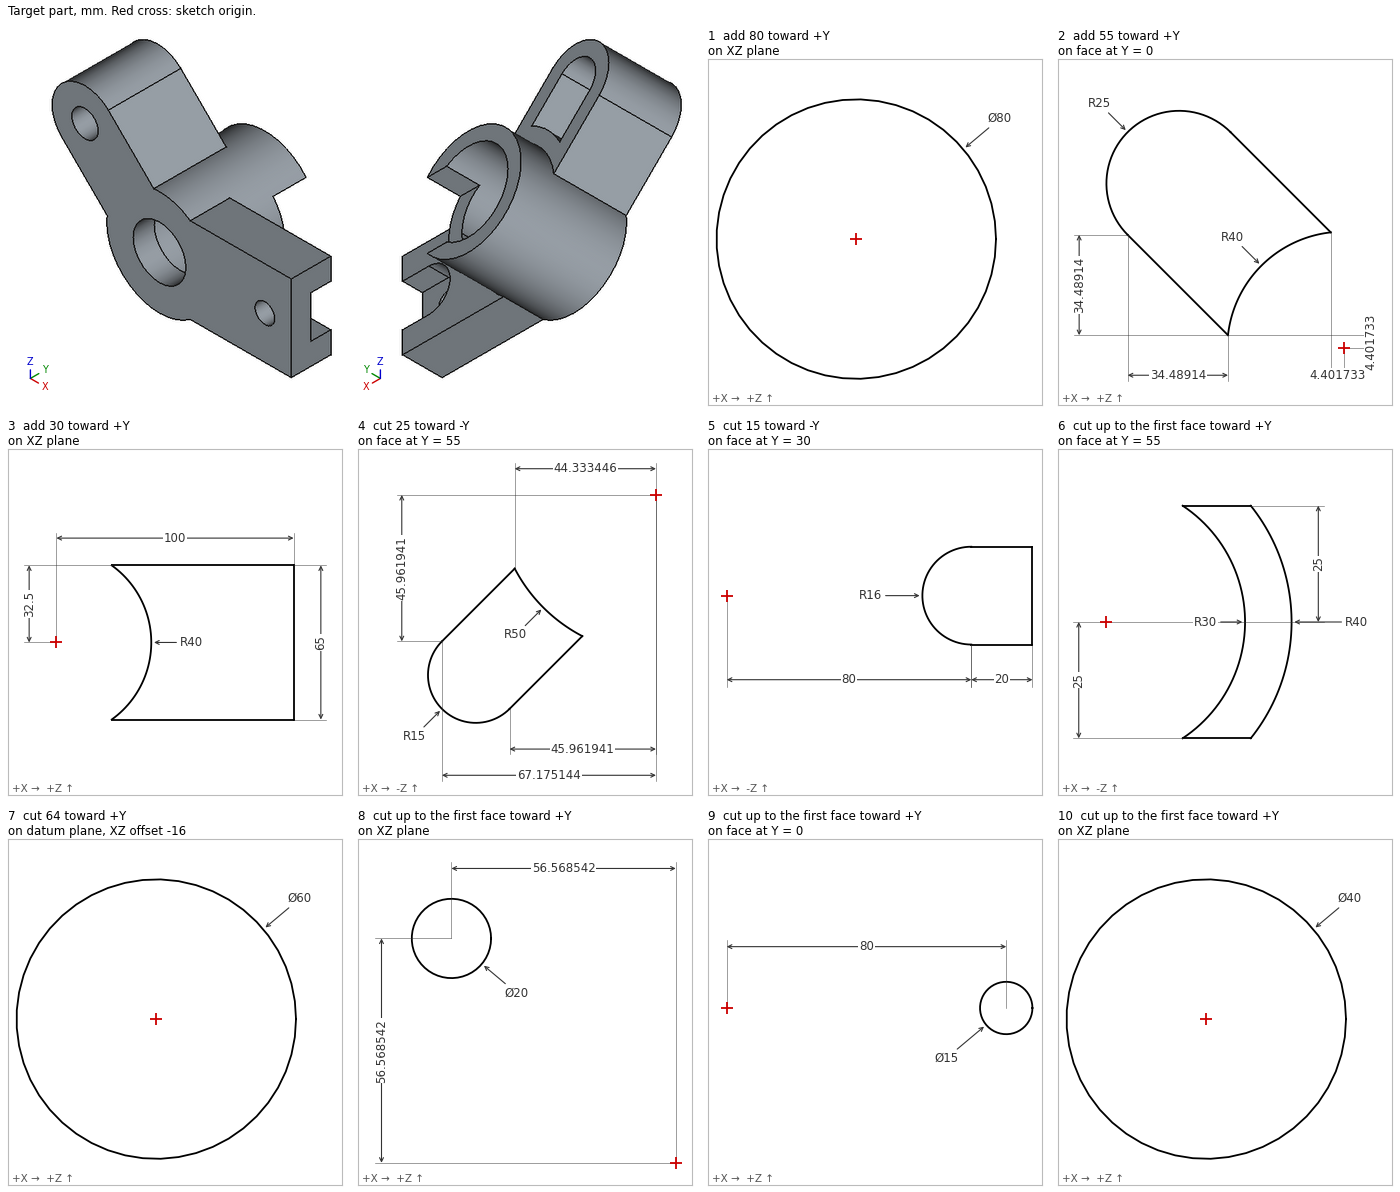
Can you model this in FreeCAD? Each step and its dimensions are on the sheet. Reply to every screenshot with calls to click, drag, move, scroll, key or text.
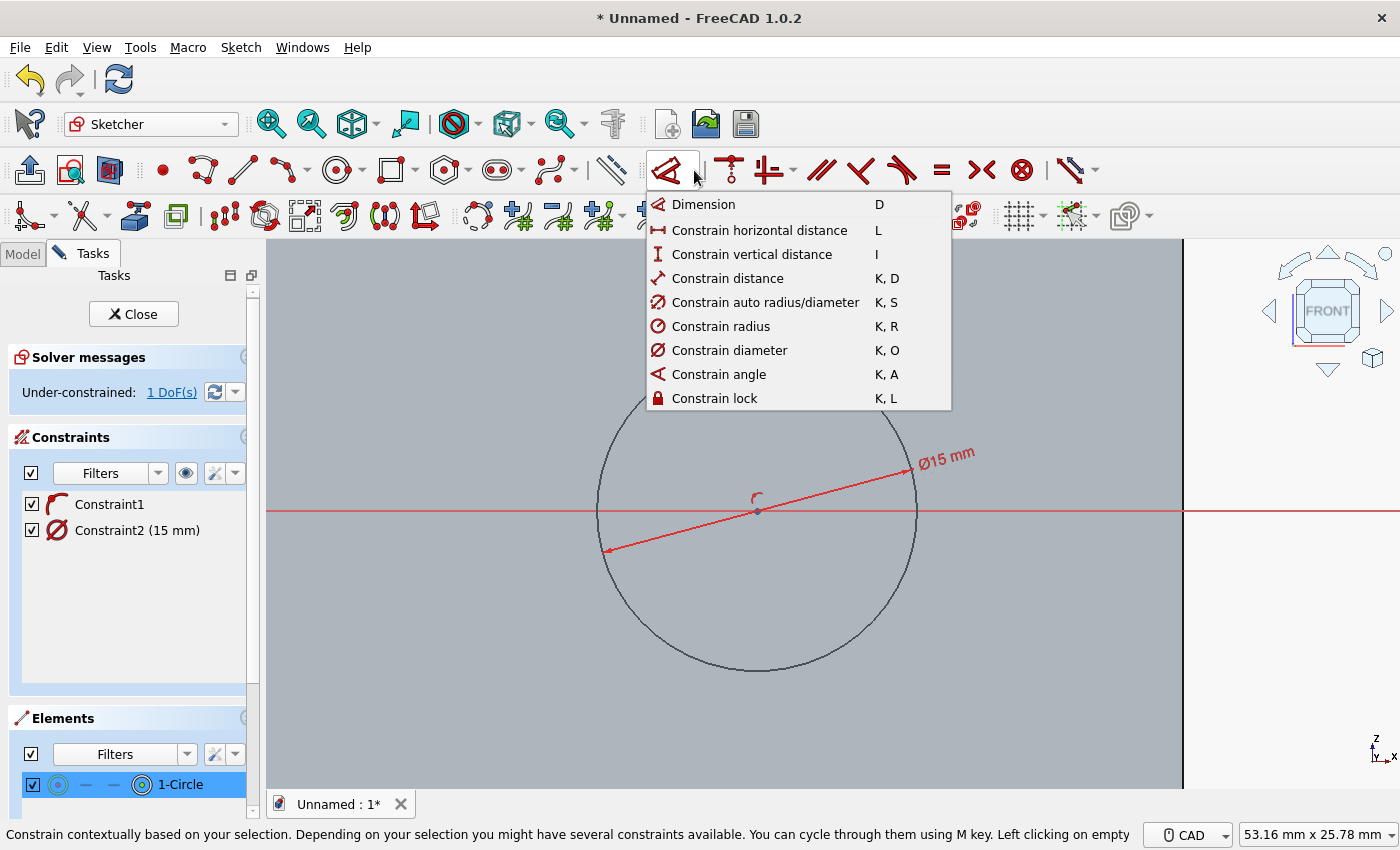
click(799, 230)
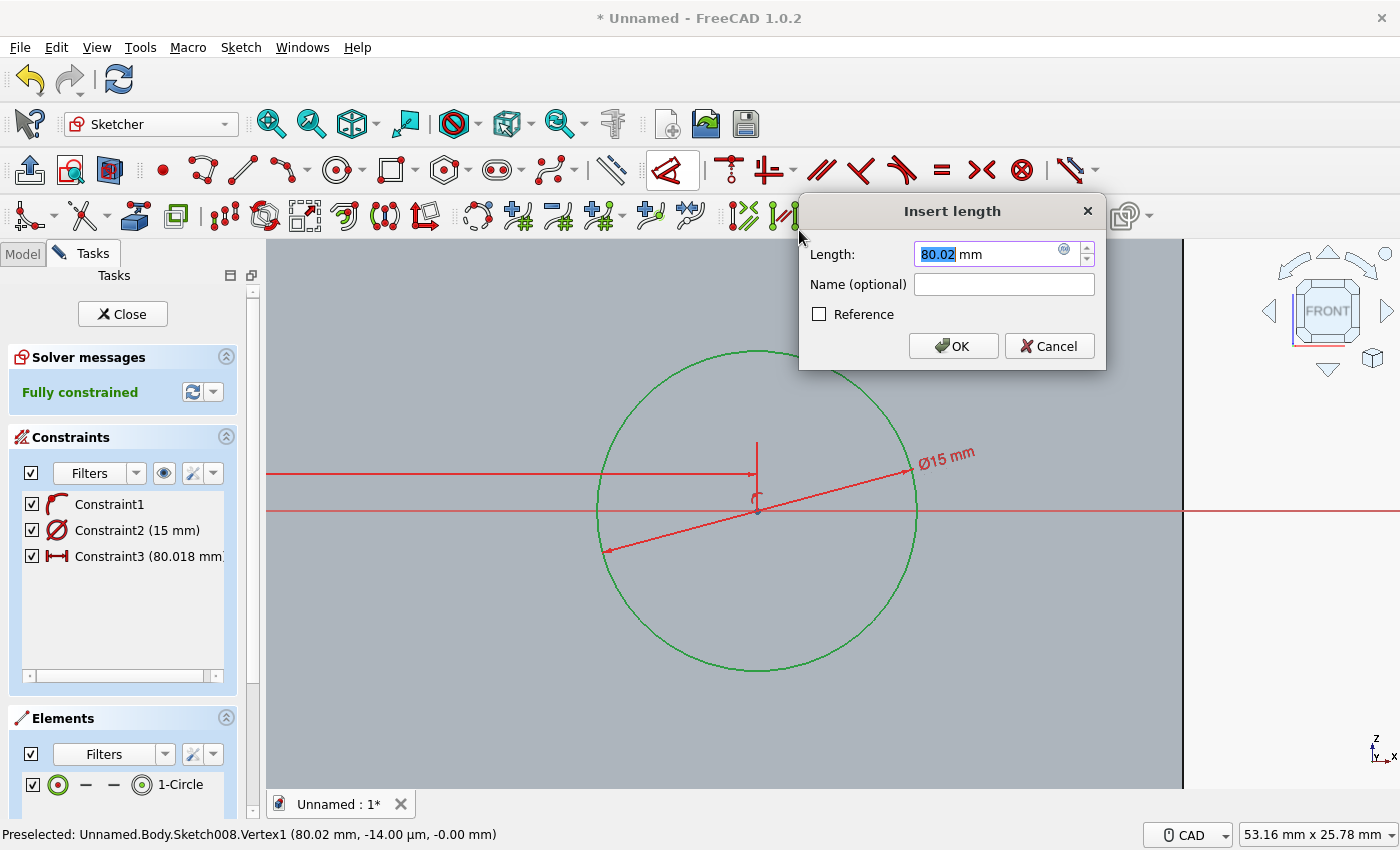
text(80)
key(Return)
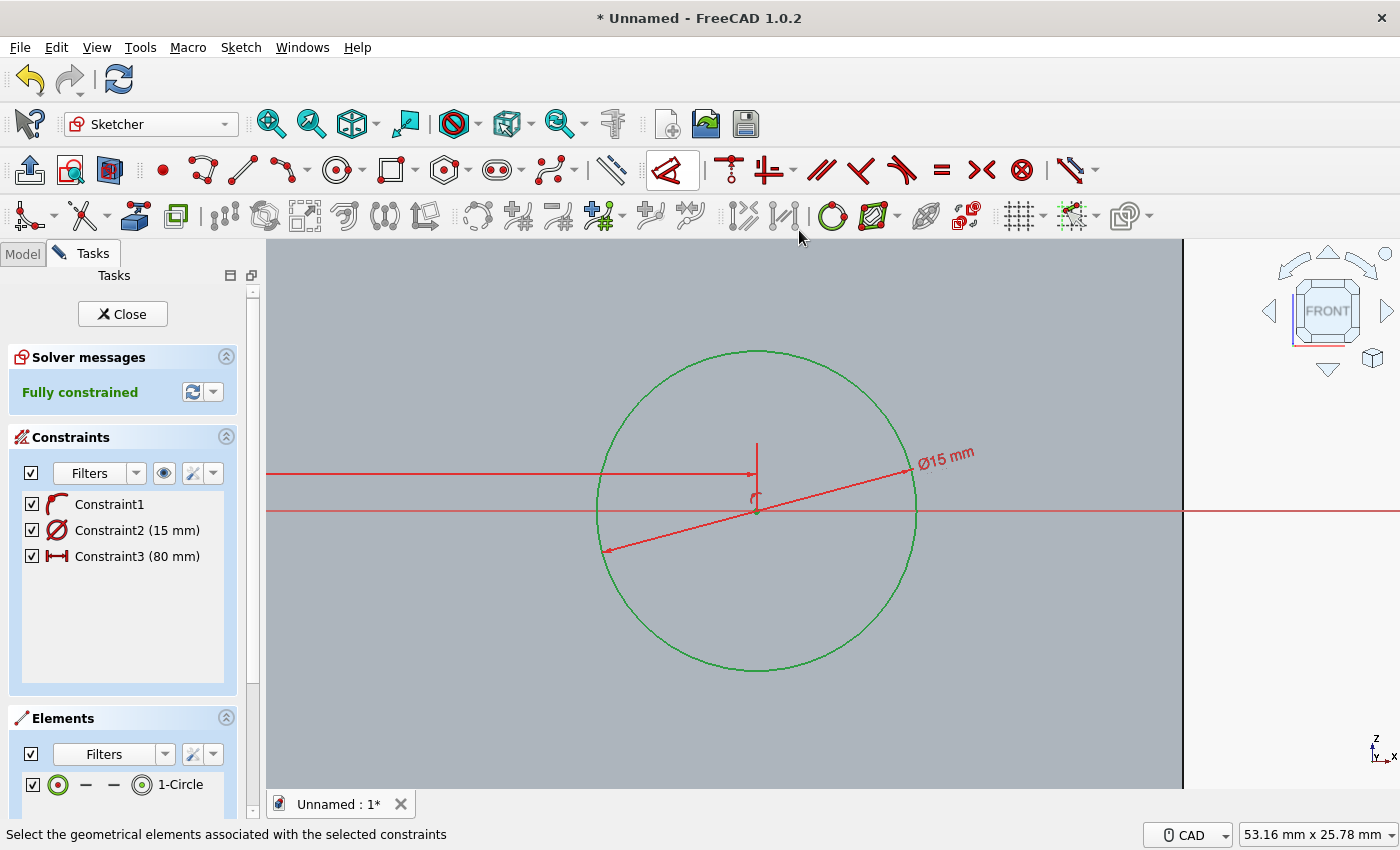
click(123, 314)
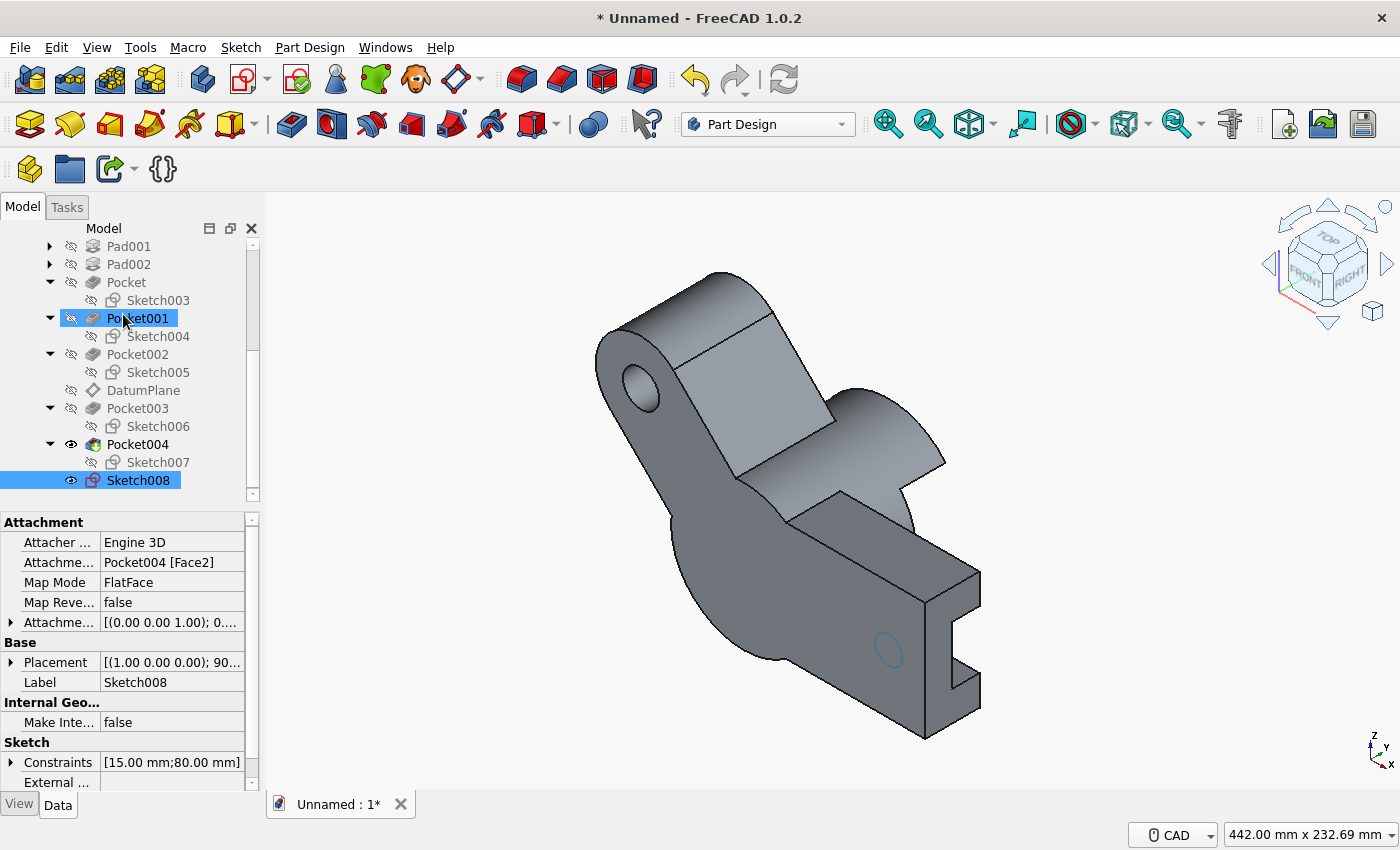
click(292, 124)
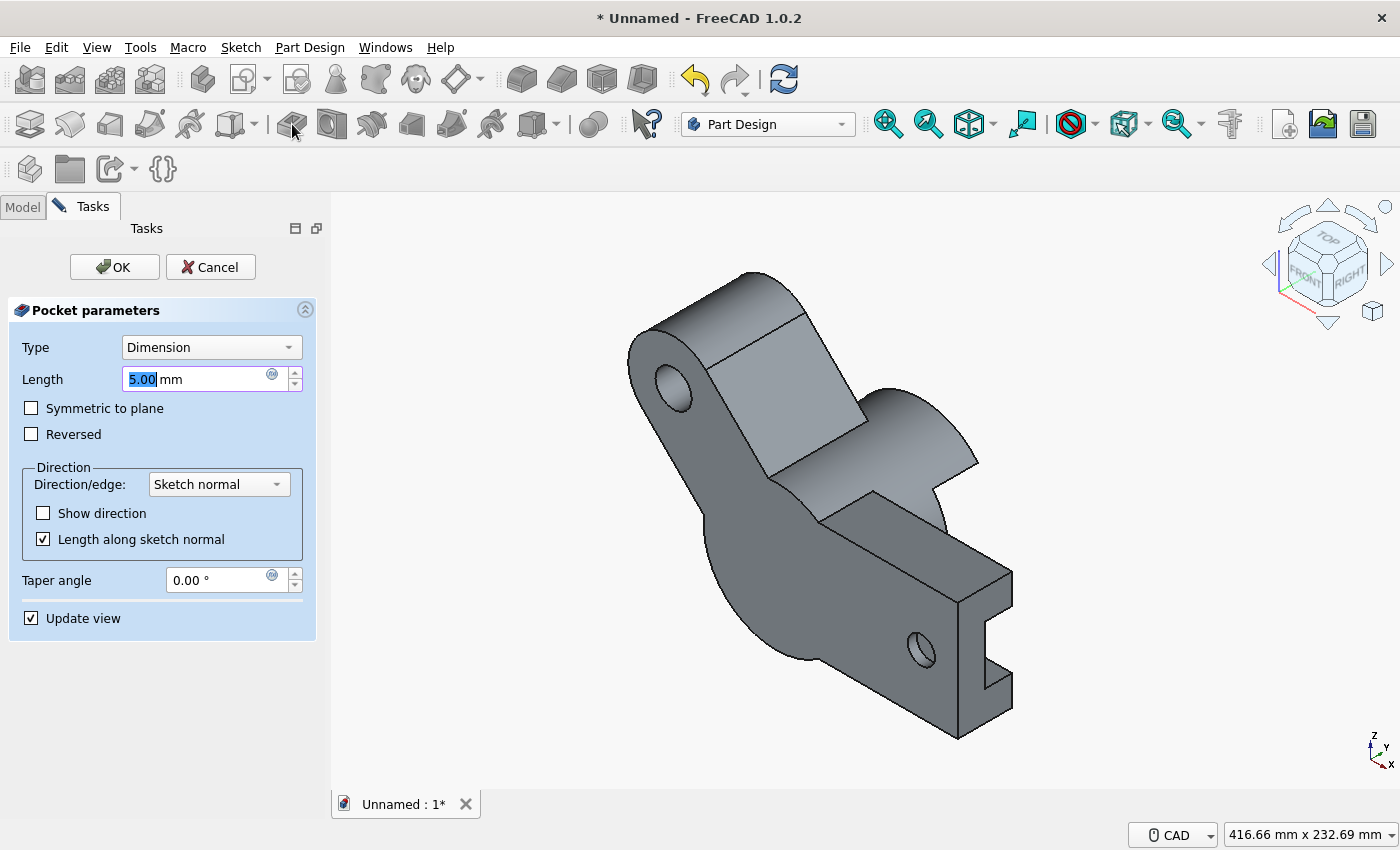
click(212, 348)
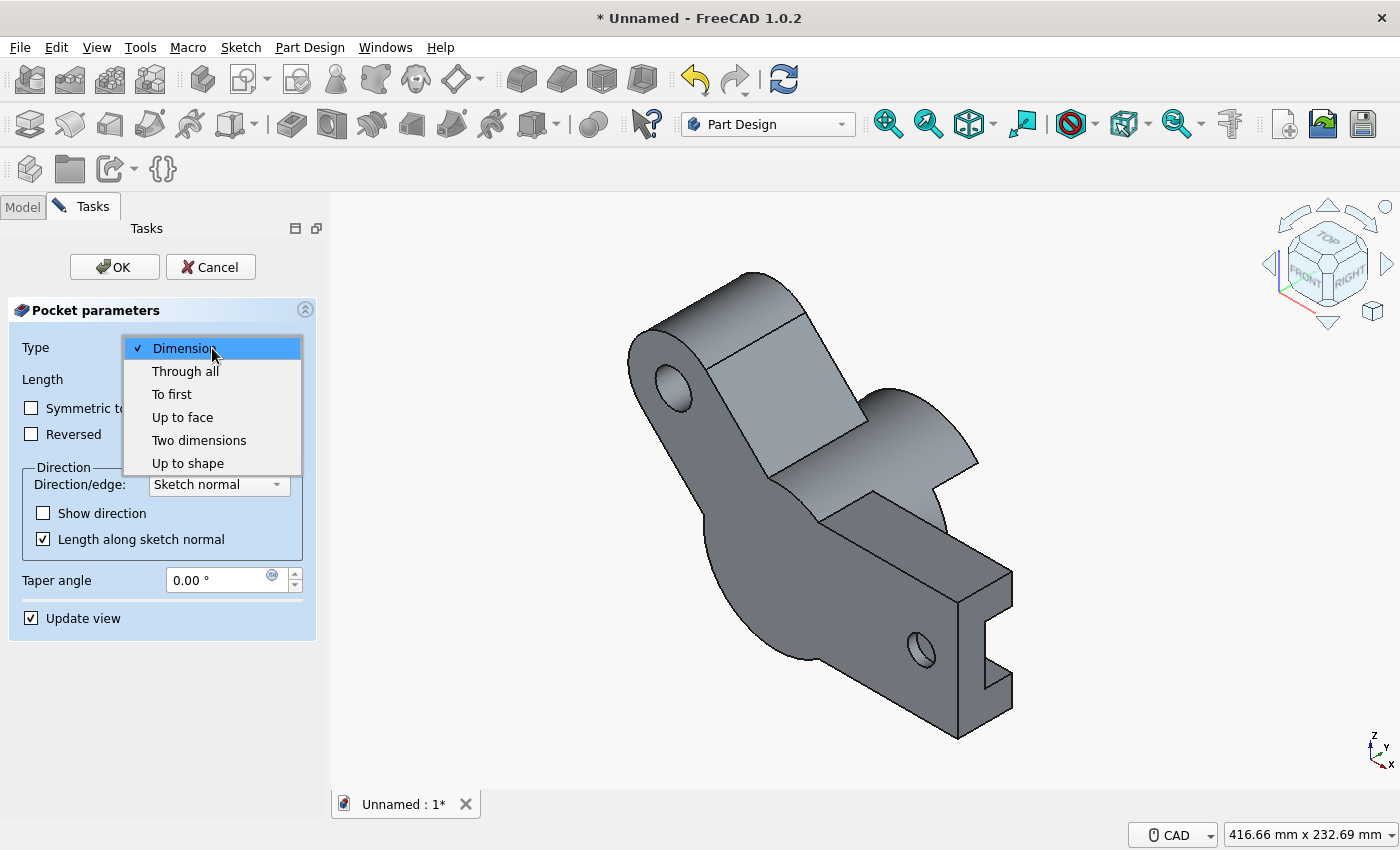
click(212, 394)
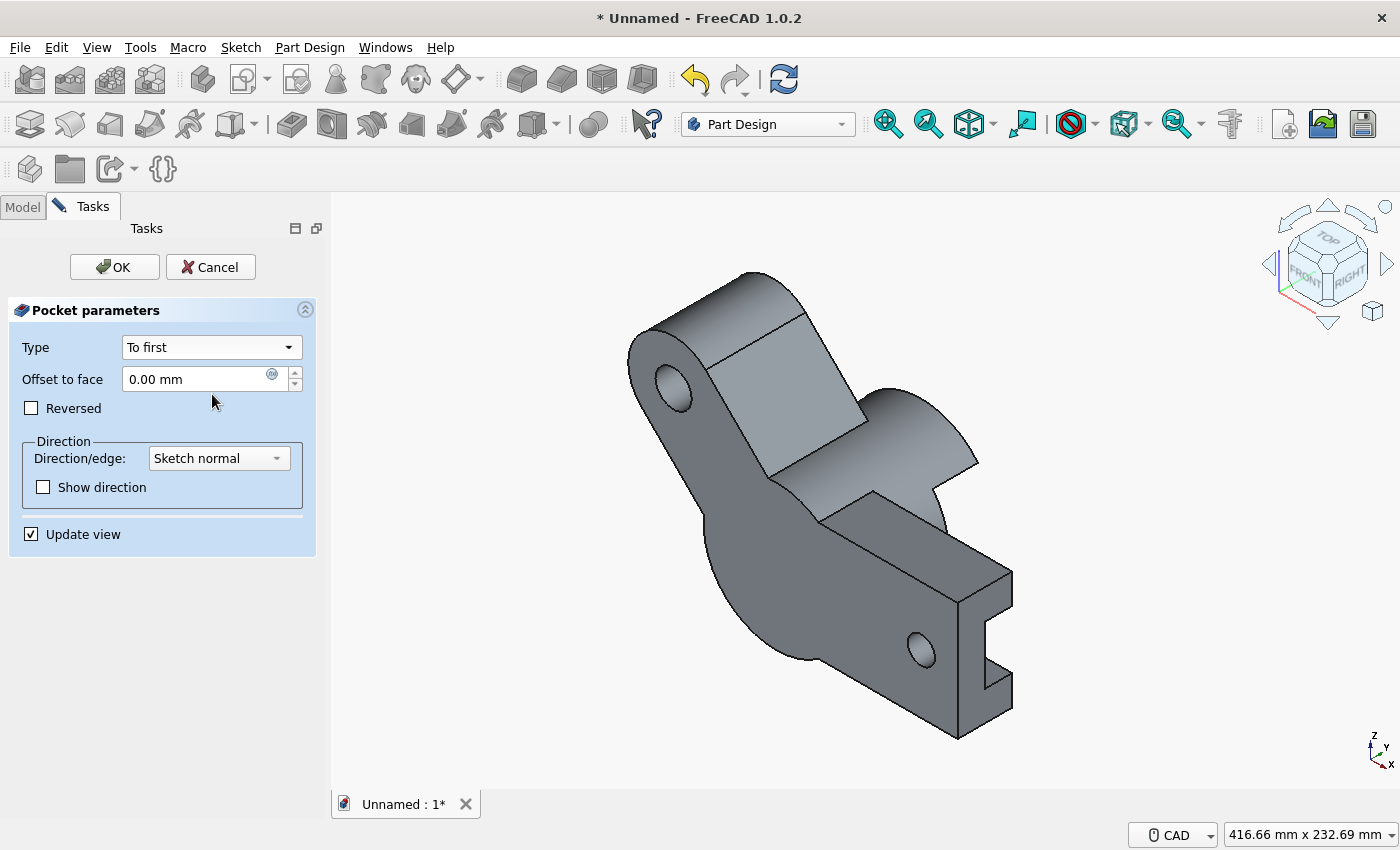
click(115, 267)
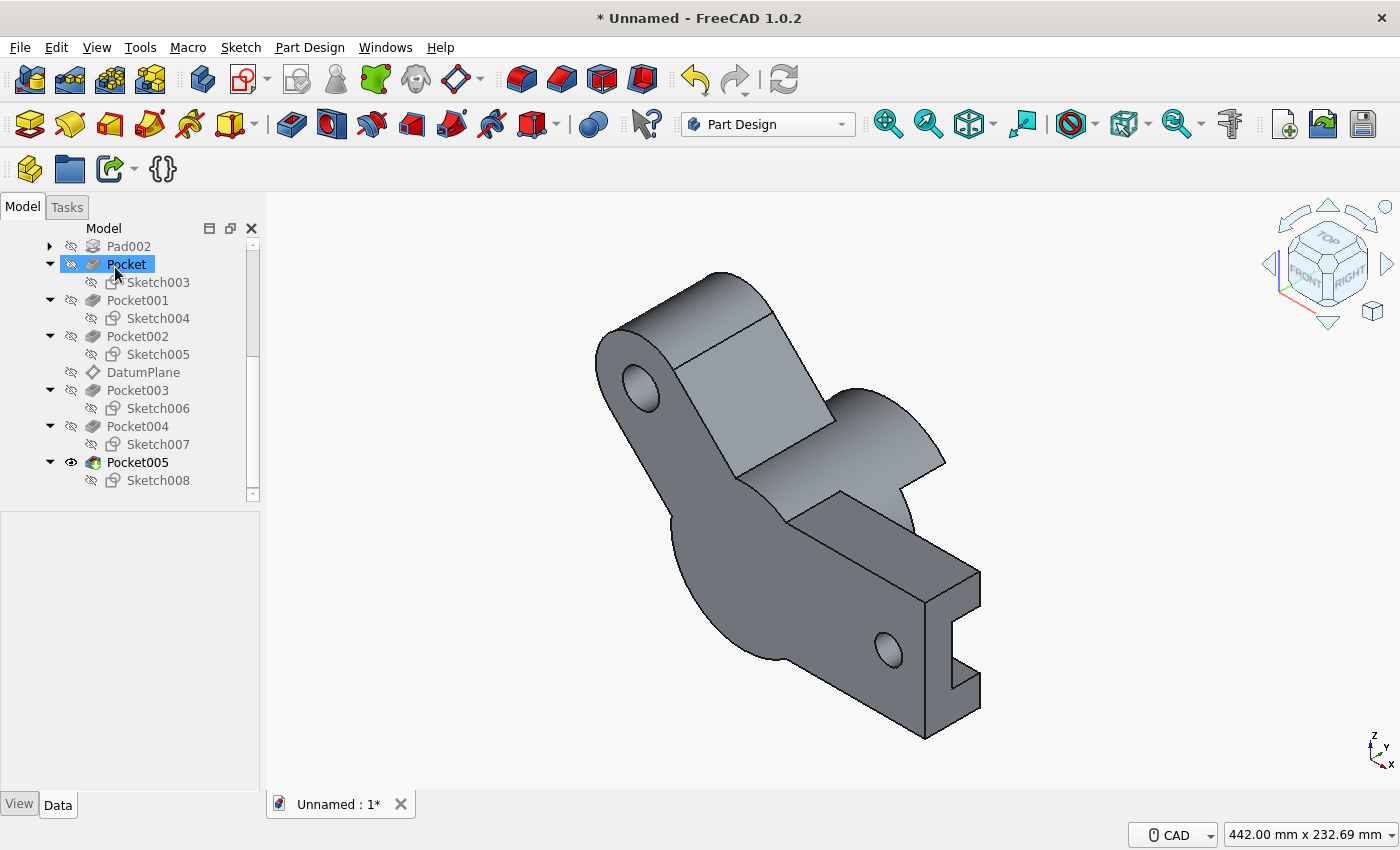
click(244, 80)